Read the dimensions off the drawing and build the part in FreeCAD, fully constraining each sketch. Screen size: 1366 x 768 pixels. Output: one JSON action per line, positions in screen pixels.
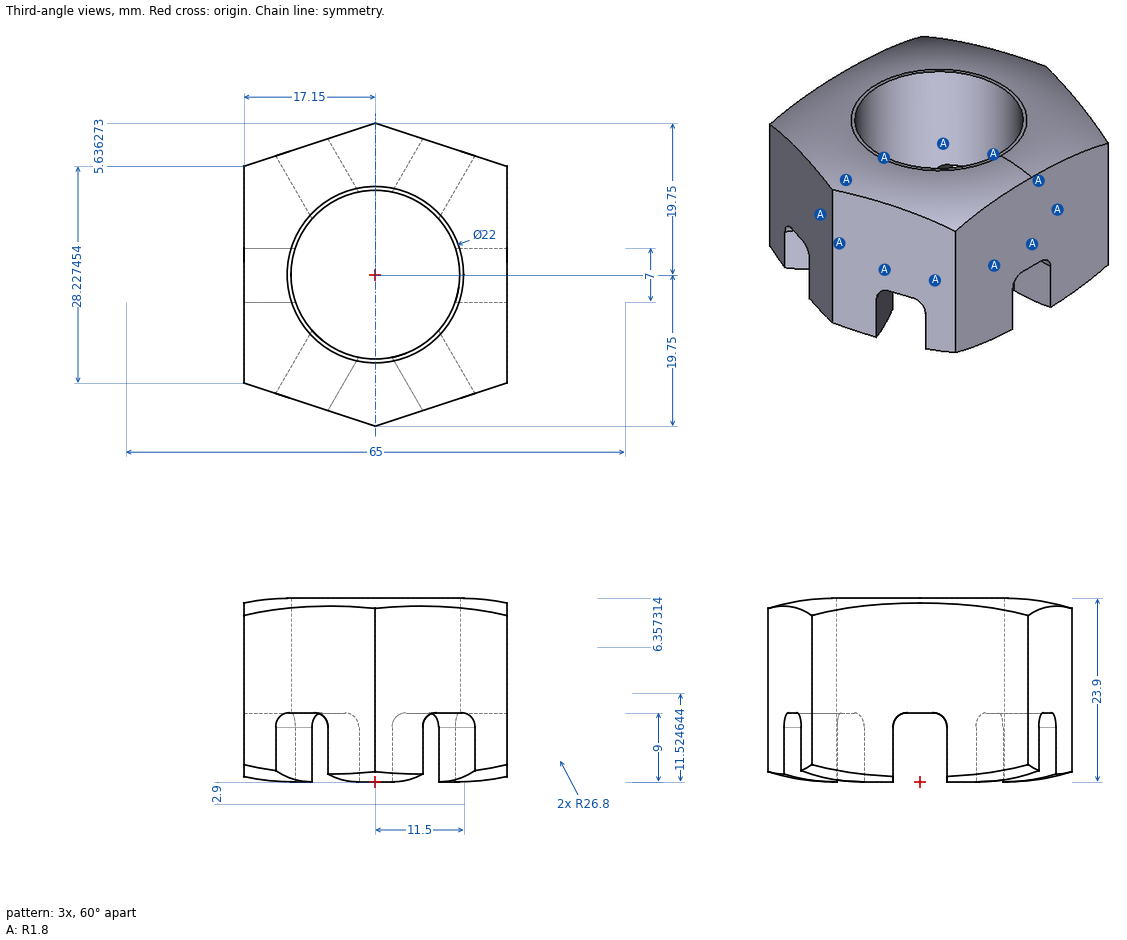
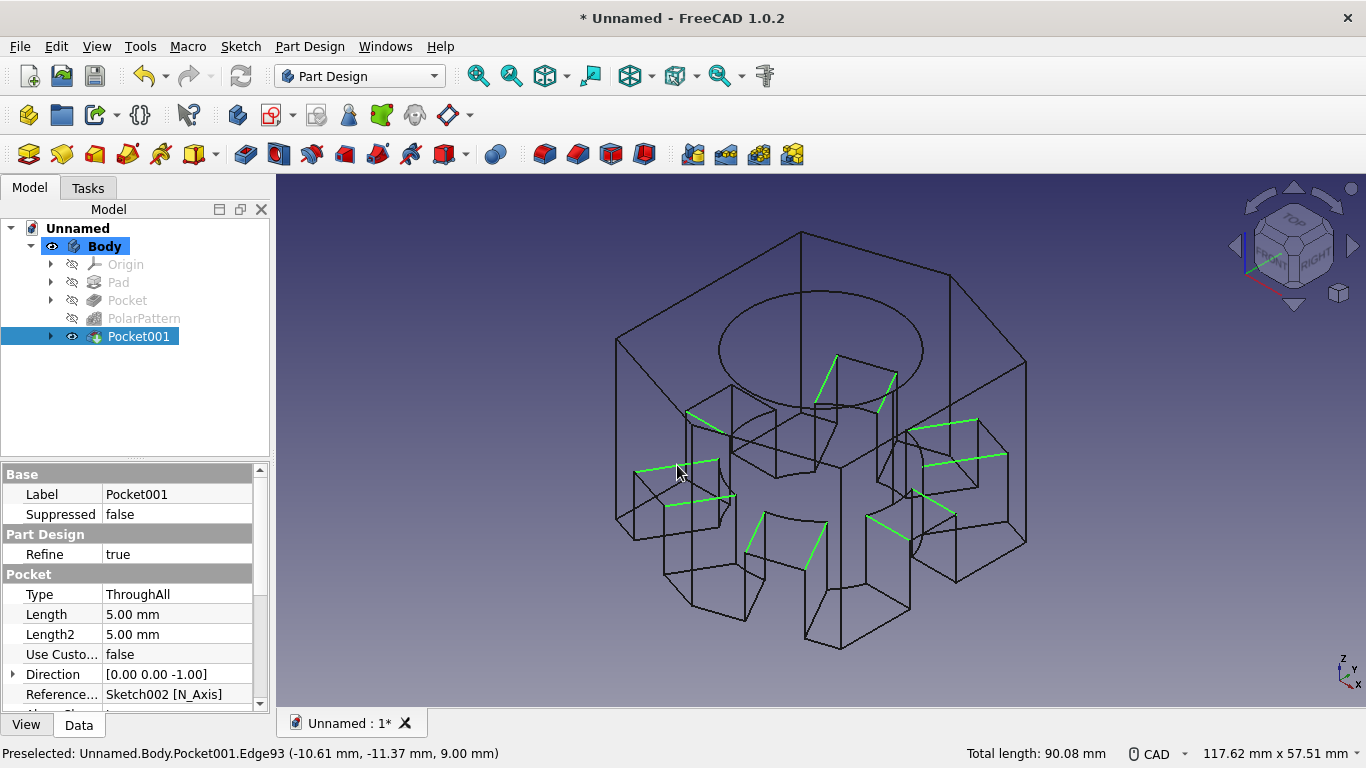
{"action": "key", "text": "2"}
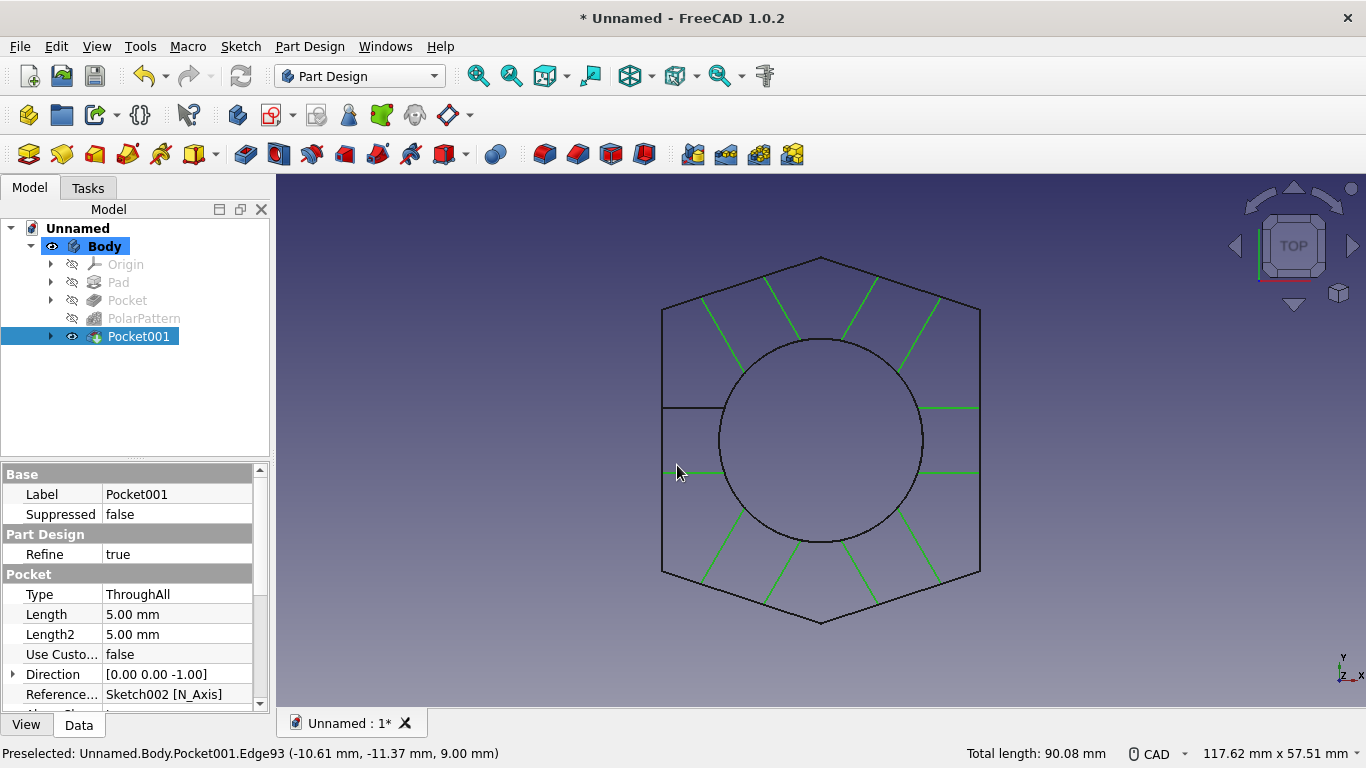
{"action": "left_click", "coordinate": [693, 407], "text": "ctrl"}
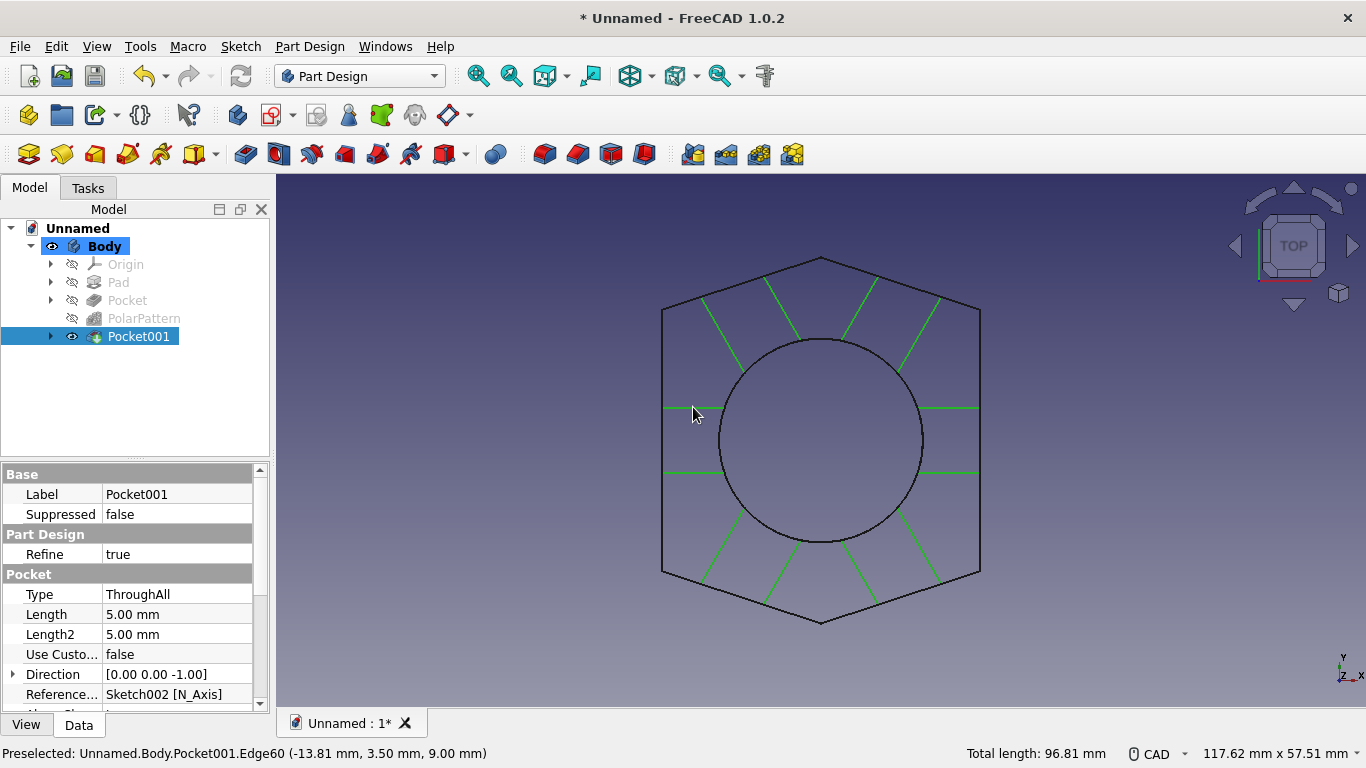
{"action": "key", "text": "v 1"}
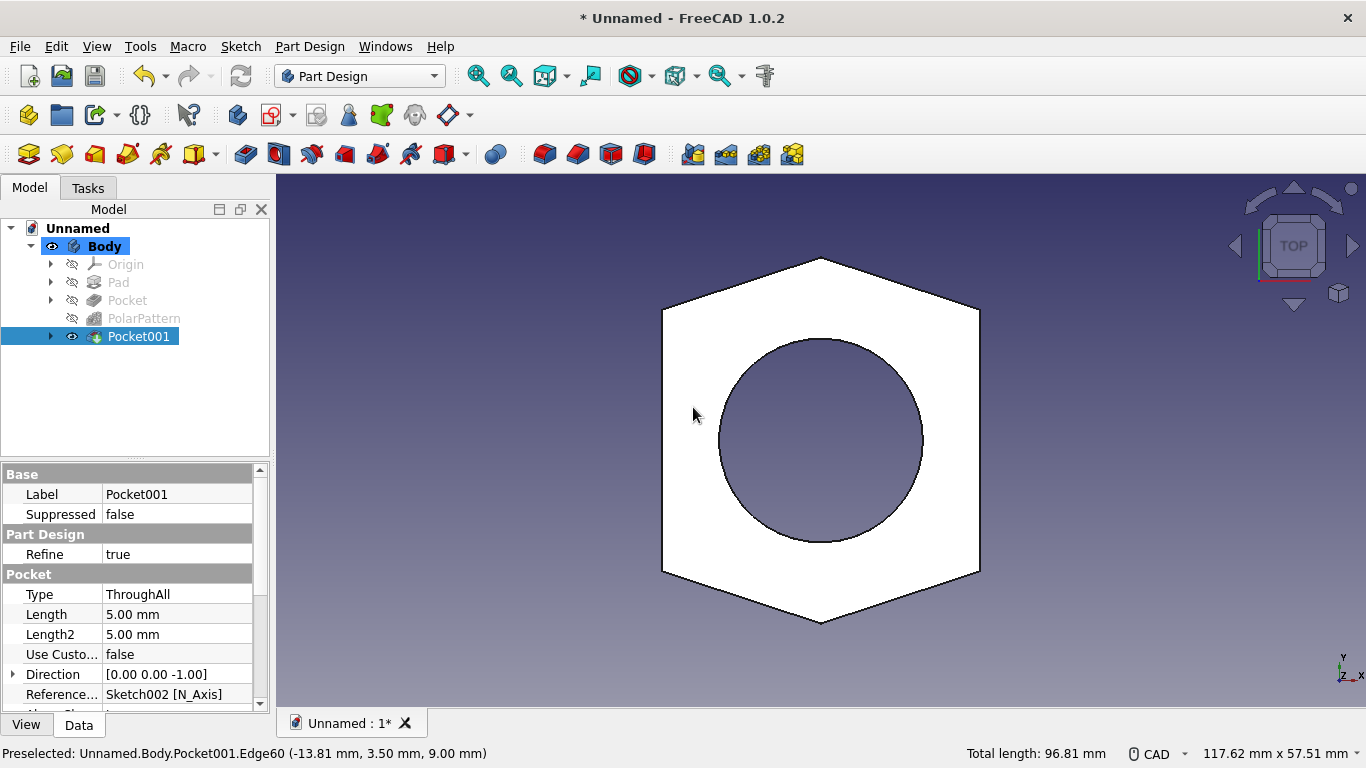
{"action": "left_click", "coordinate": [545, 154]}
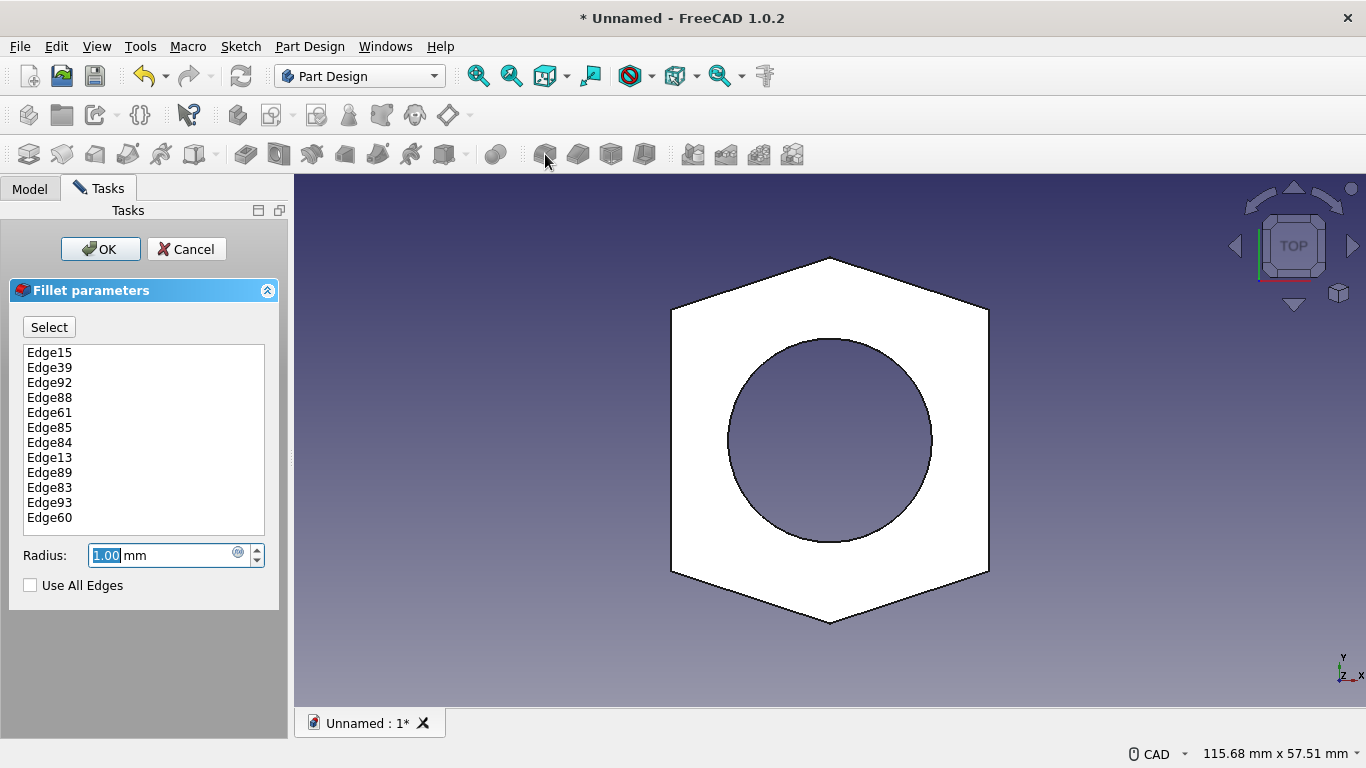
{"action": "type", "text": "1.8"}
{"action": "key", "text": "Tab"}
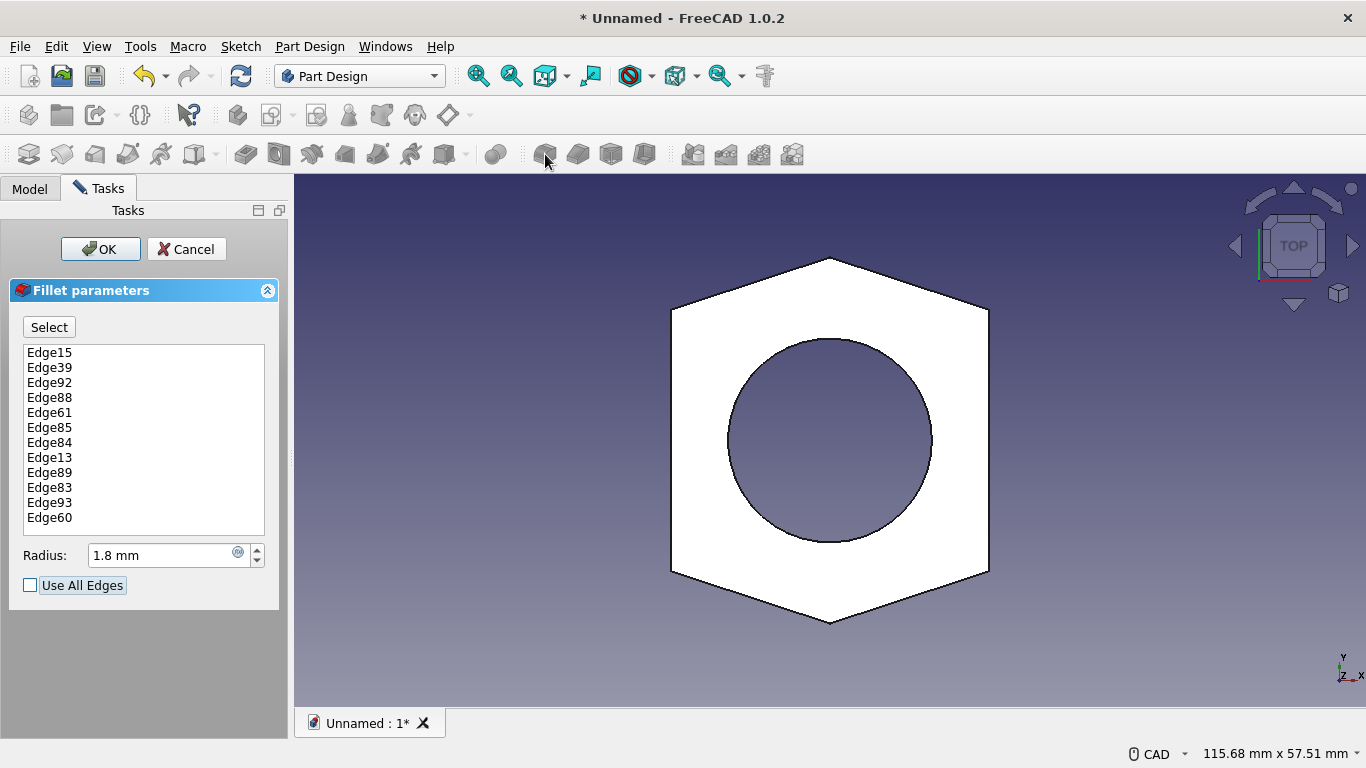
{"action": "left_click", "coordinate": [101, 249]}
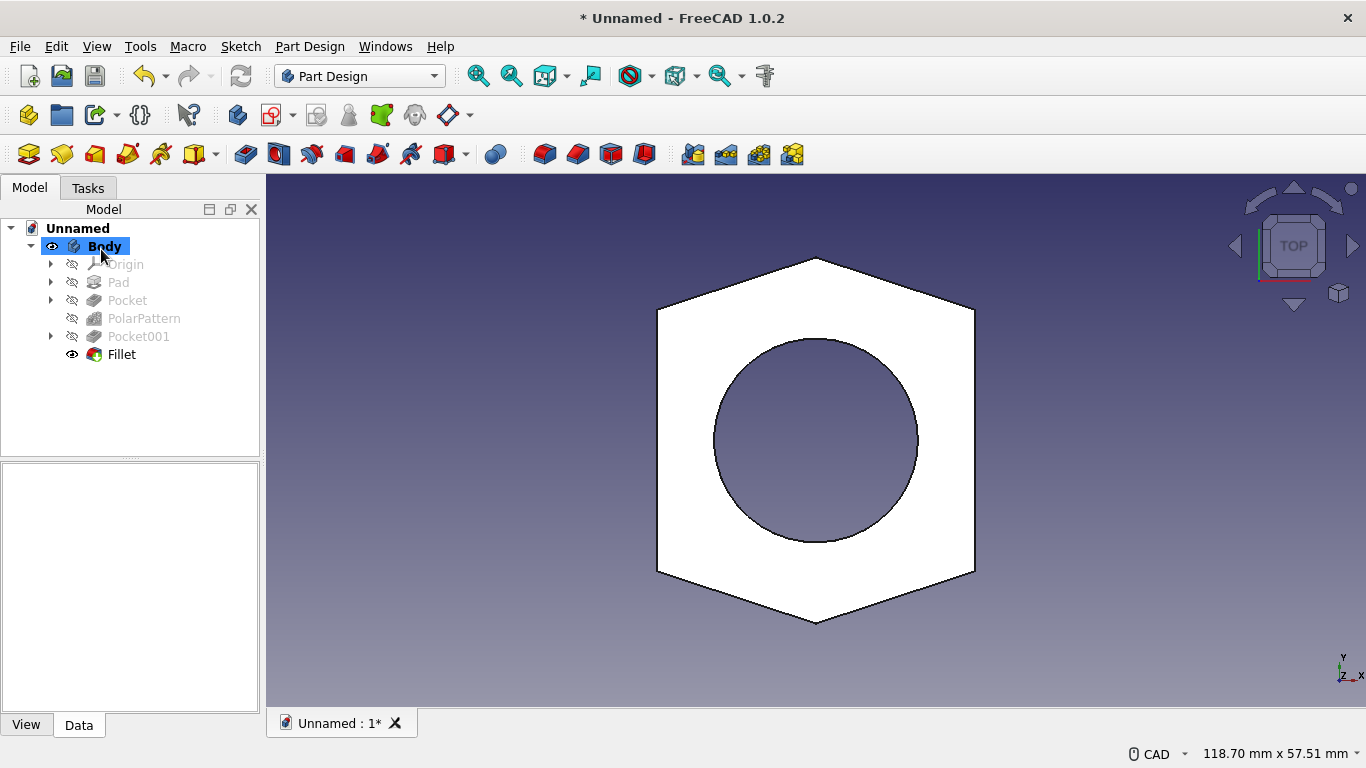
{"action": "left_click", "coordinate": [270, 116]}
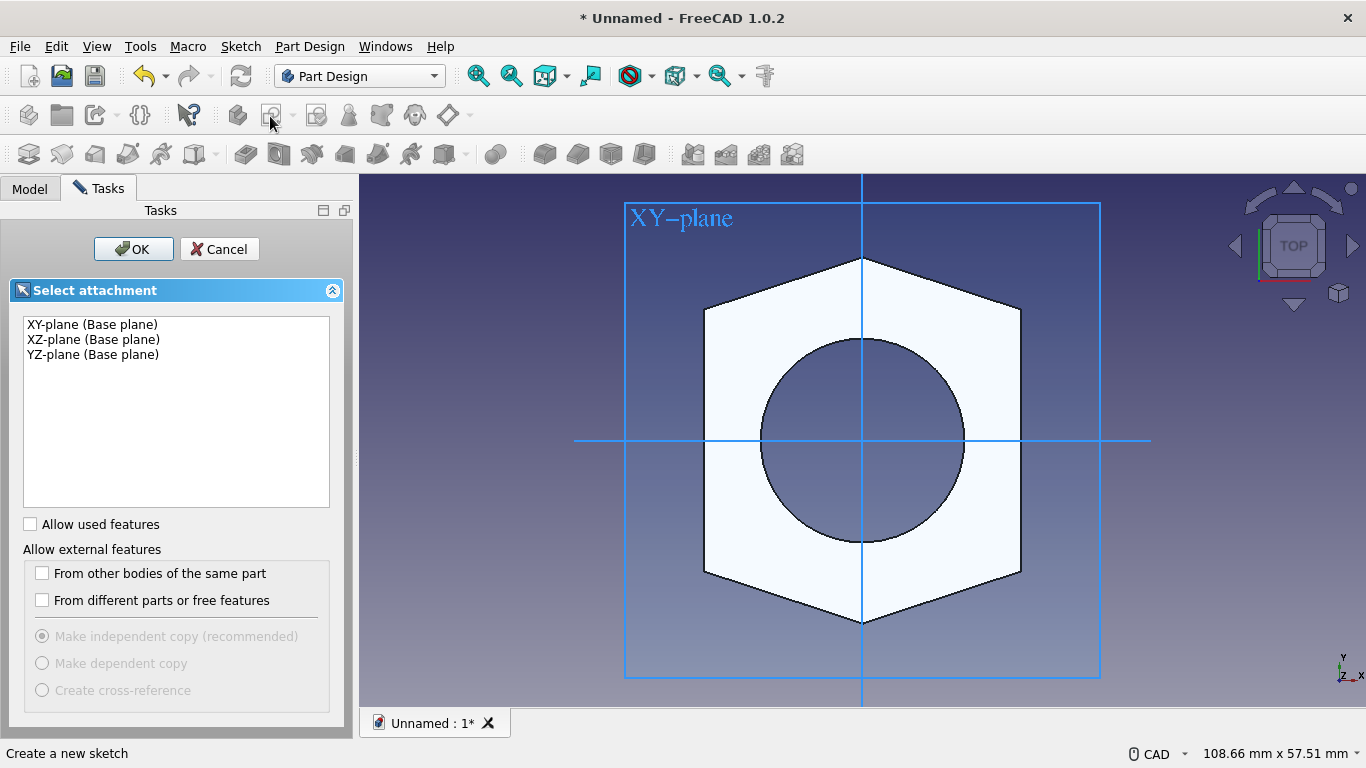
{"action": "left_click", "coordinate": [84, 340]}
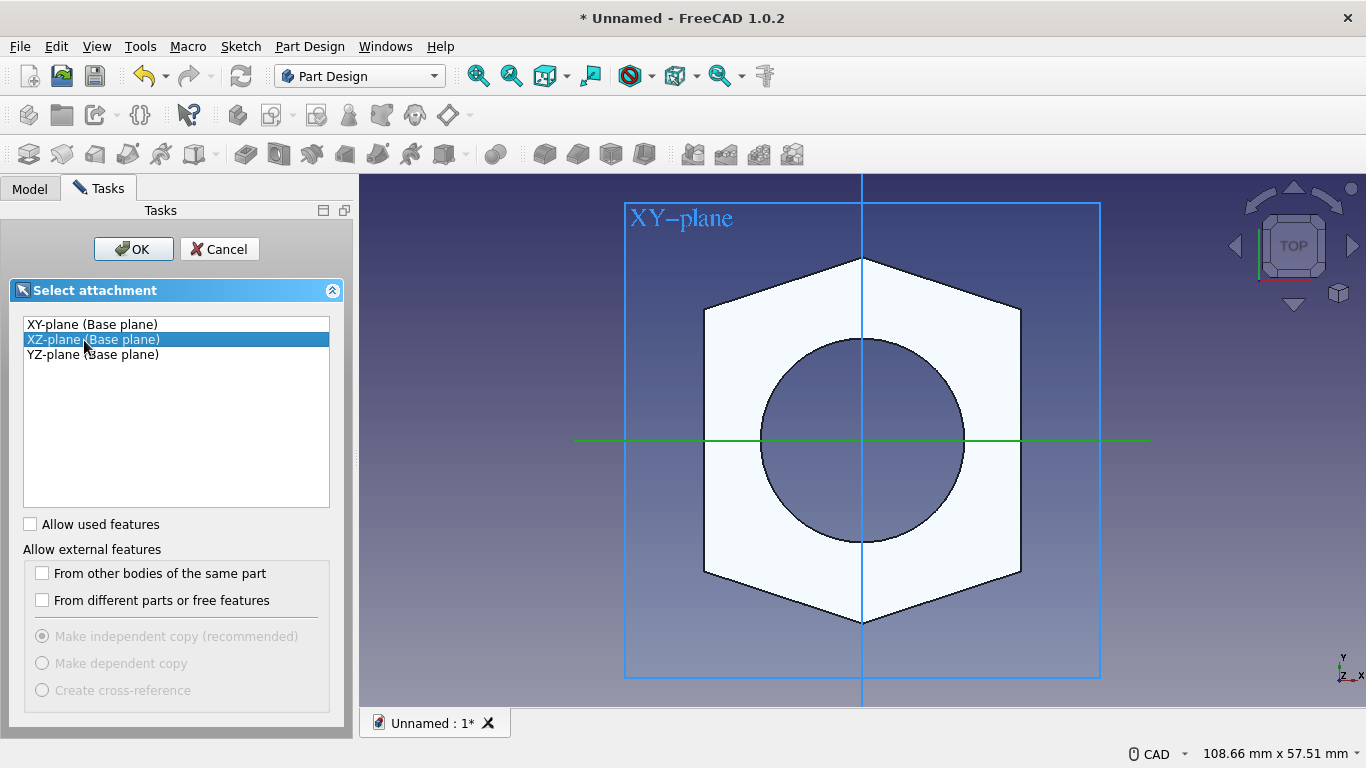
{"action": "left_click", "coordinate": [134, 249]}